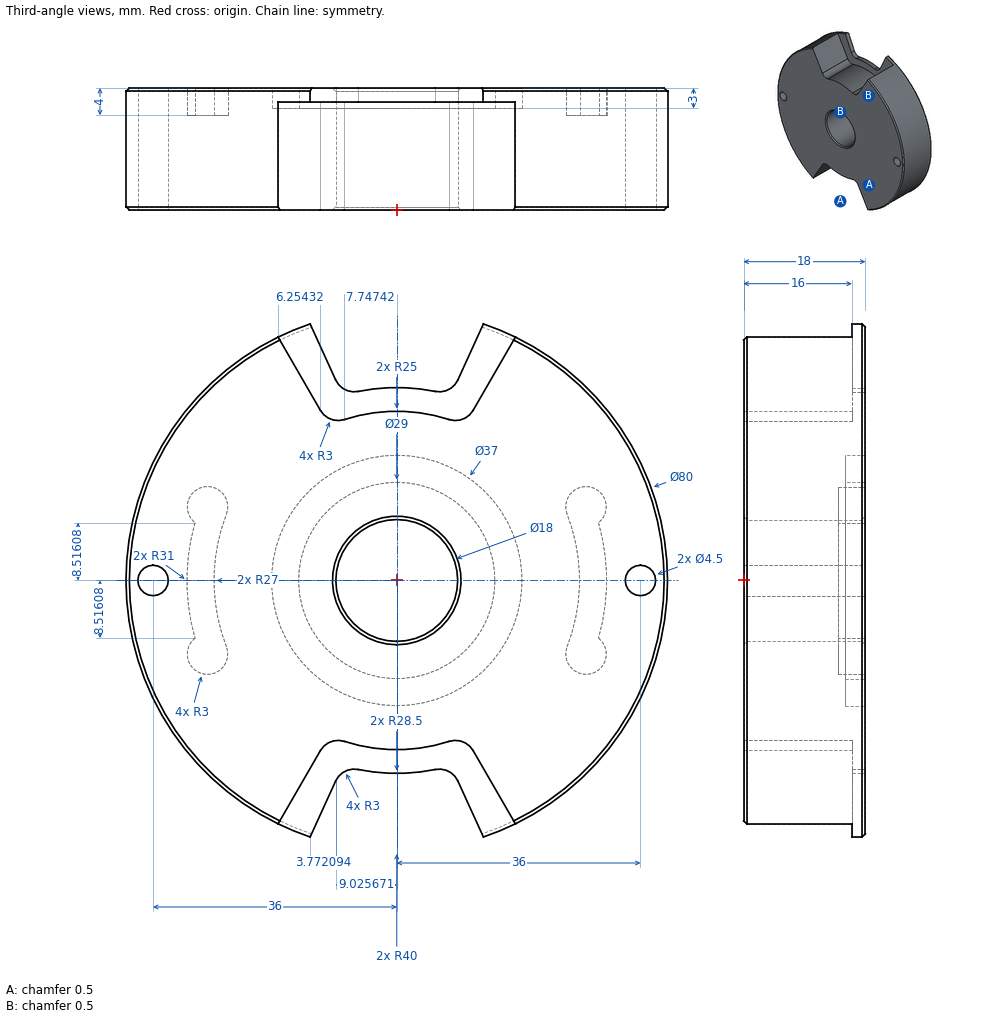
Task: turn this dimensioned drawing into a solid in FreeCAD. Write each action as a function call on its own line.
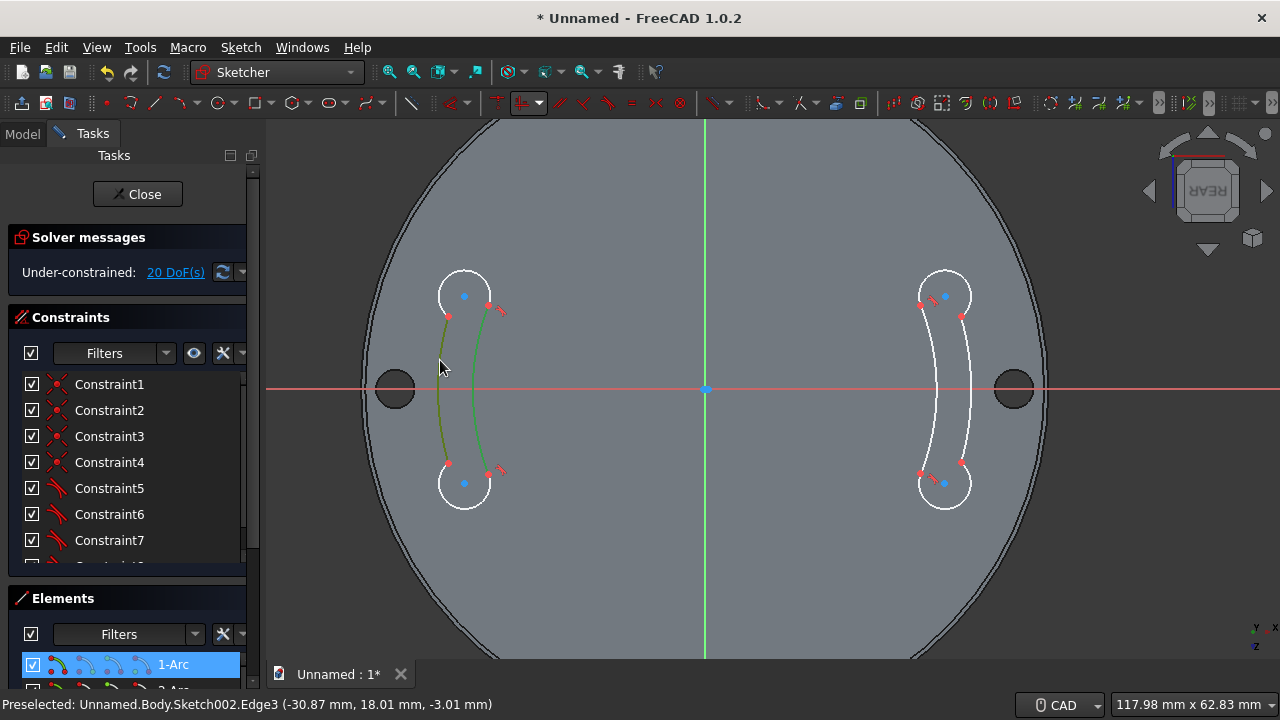
click(498, 104)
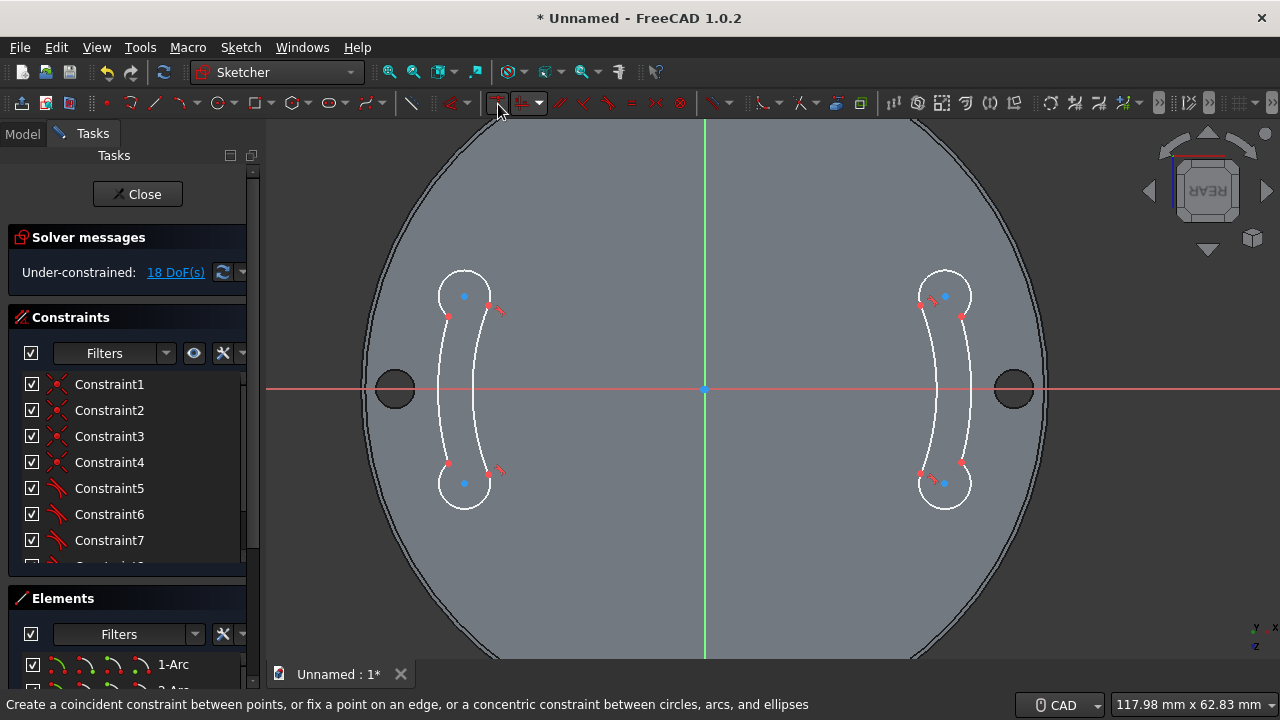
click(475, 355)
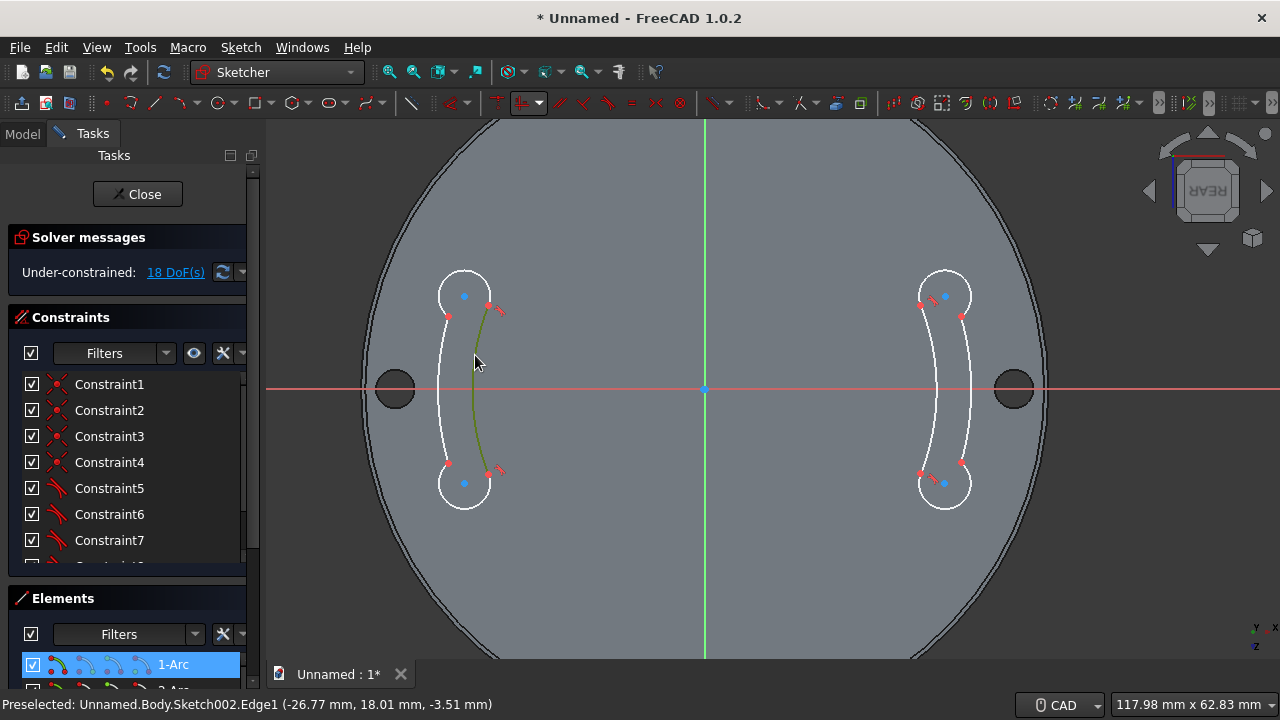
click(970, 420)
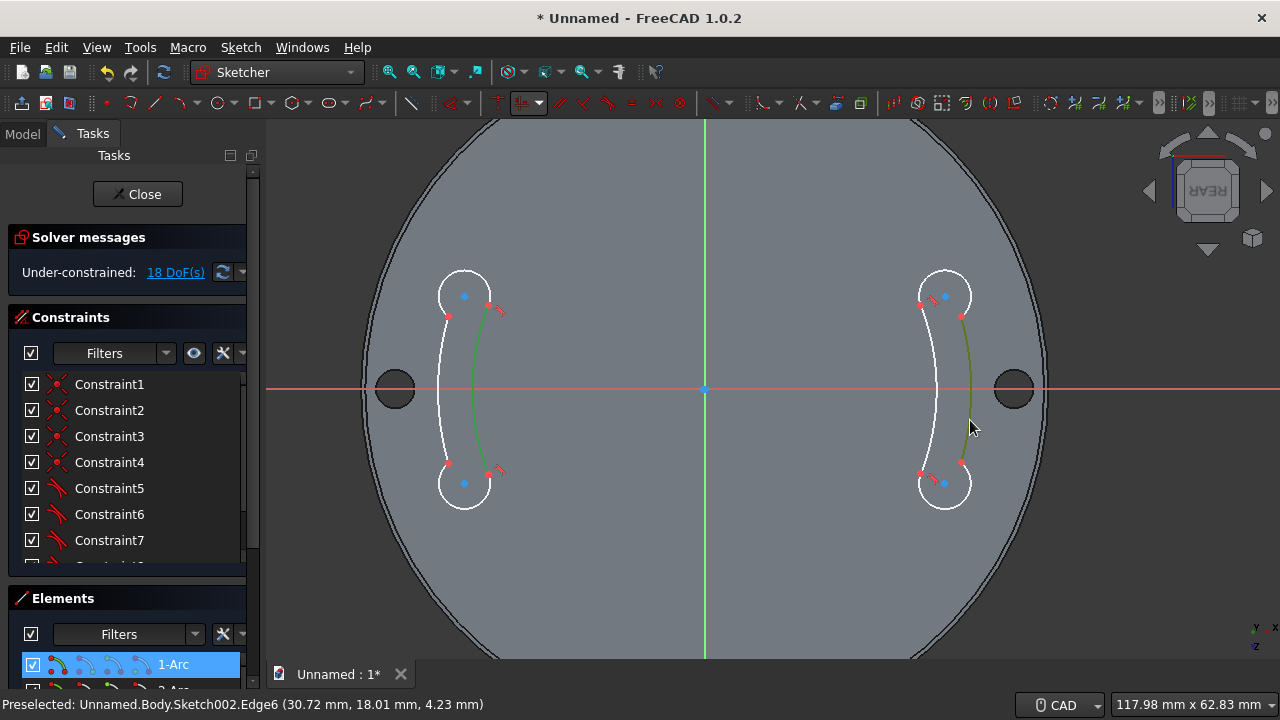
click(498, 104)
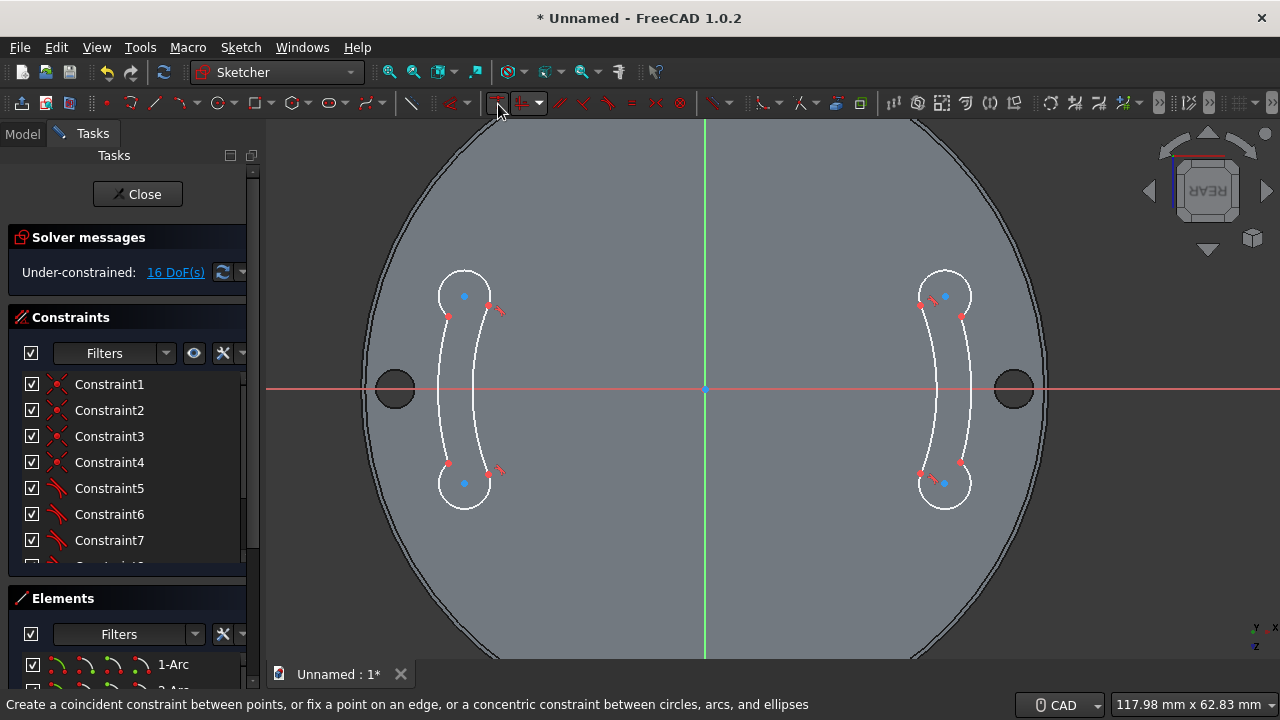
click(475, 355)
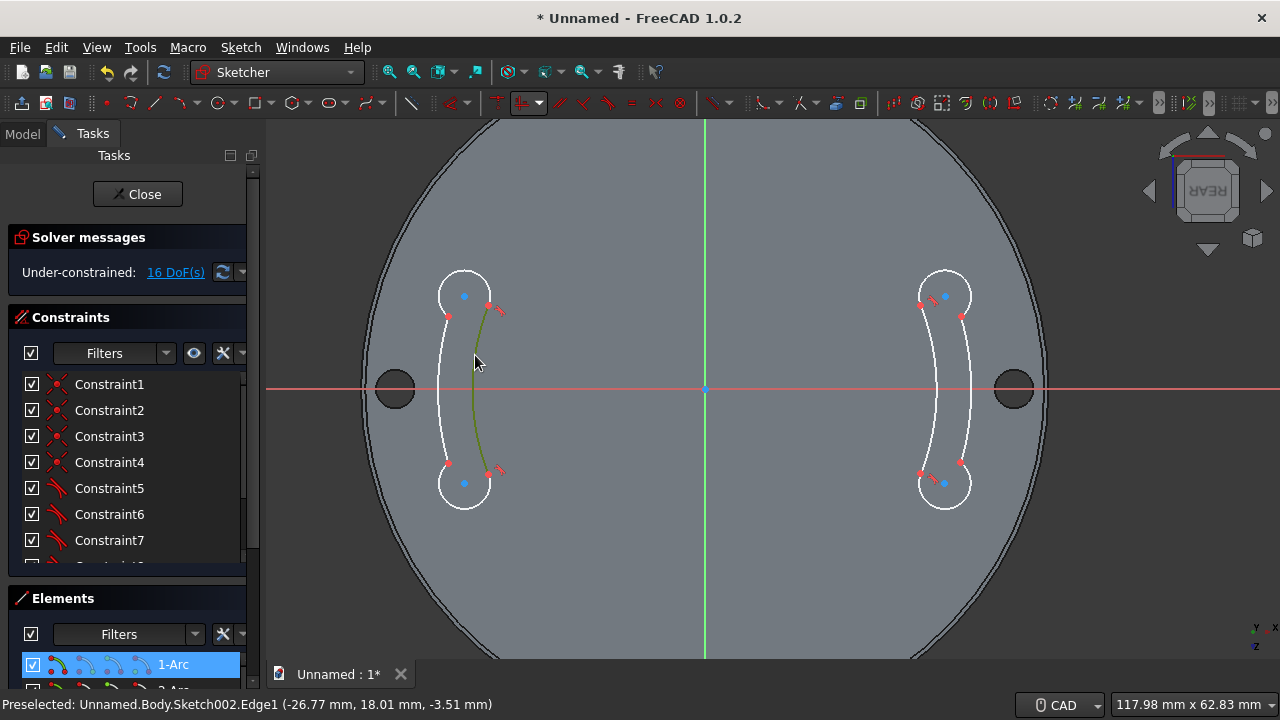
click(934, 424)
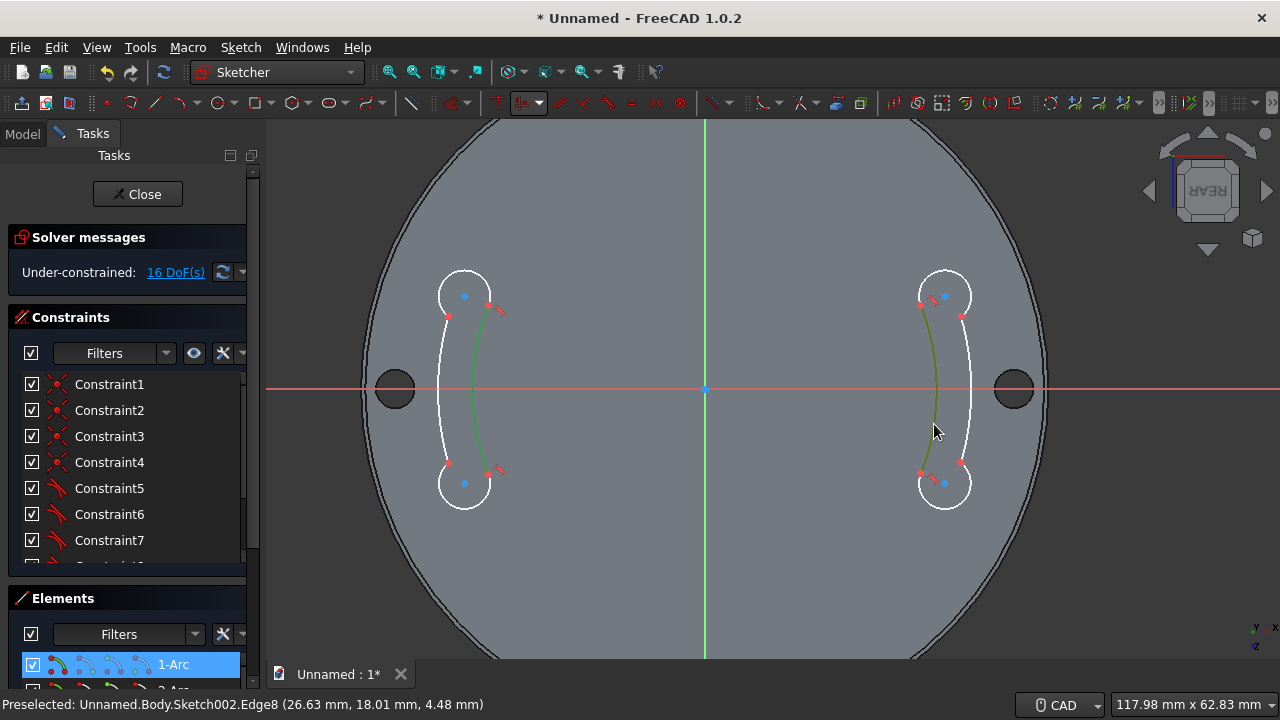
click(498, 104)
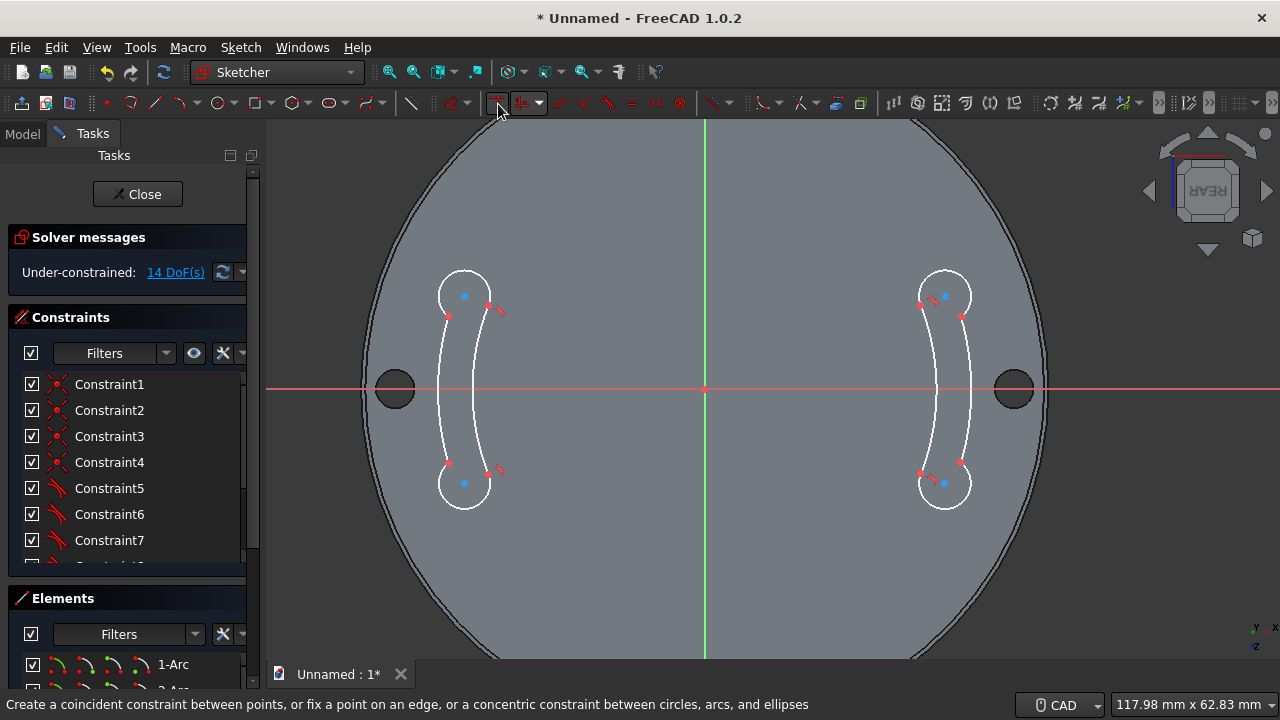
scroll(704, 389, up, 3)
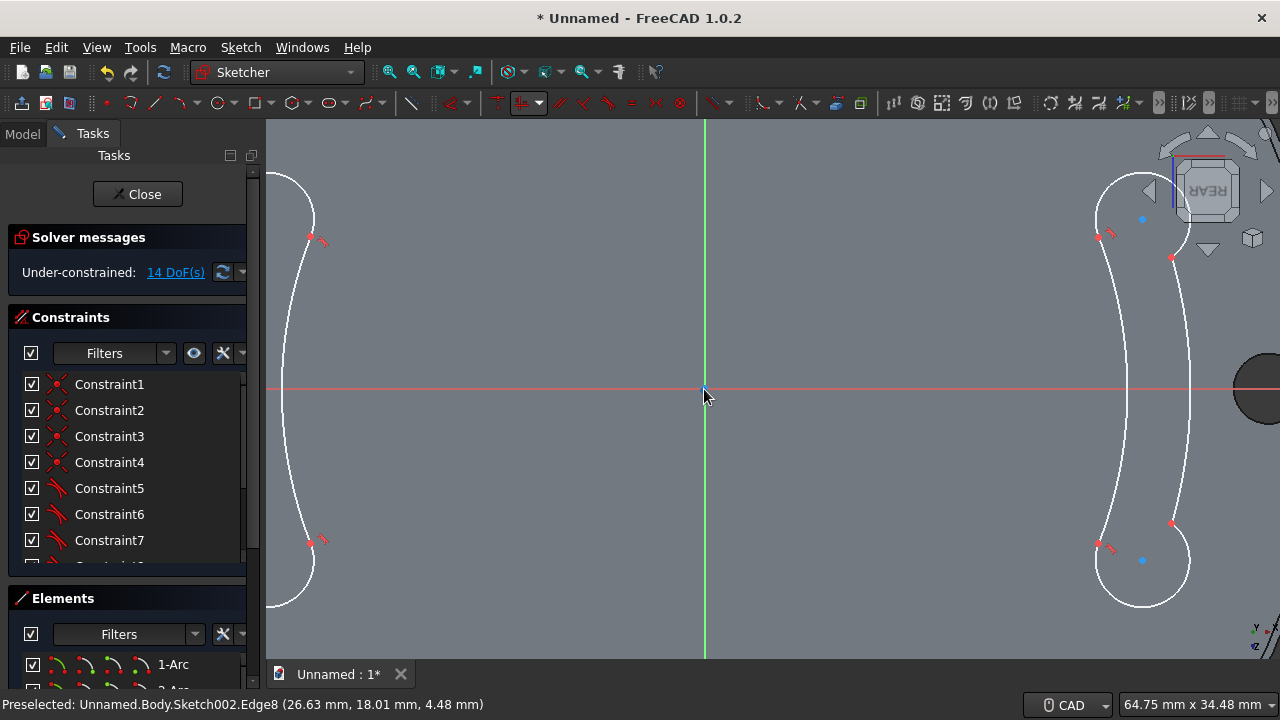
drag(694, 379, 715, 400)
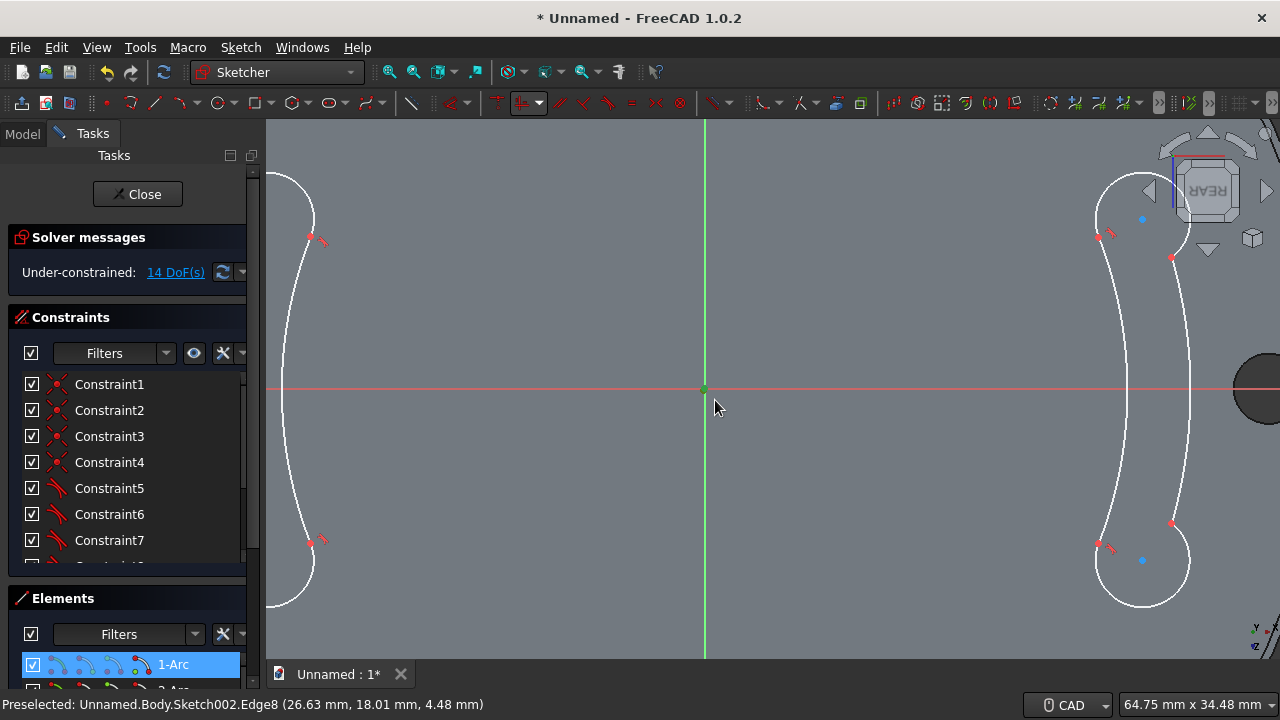
click(498, 104)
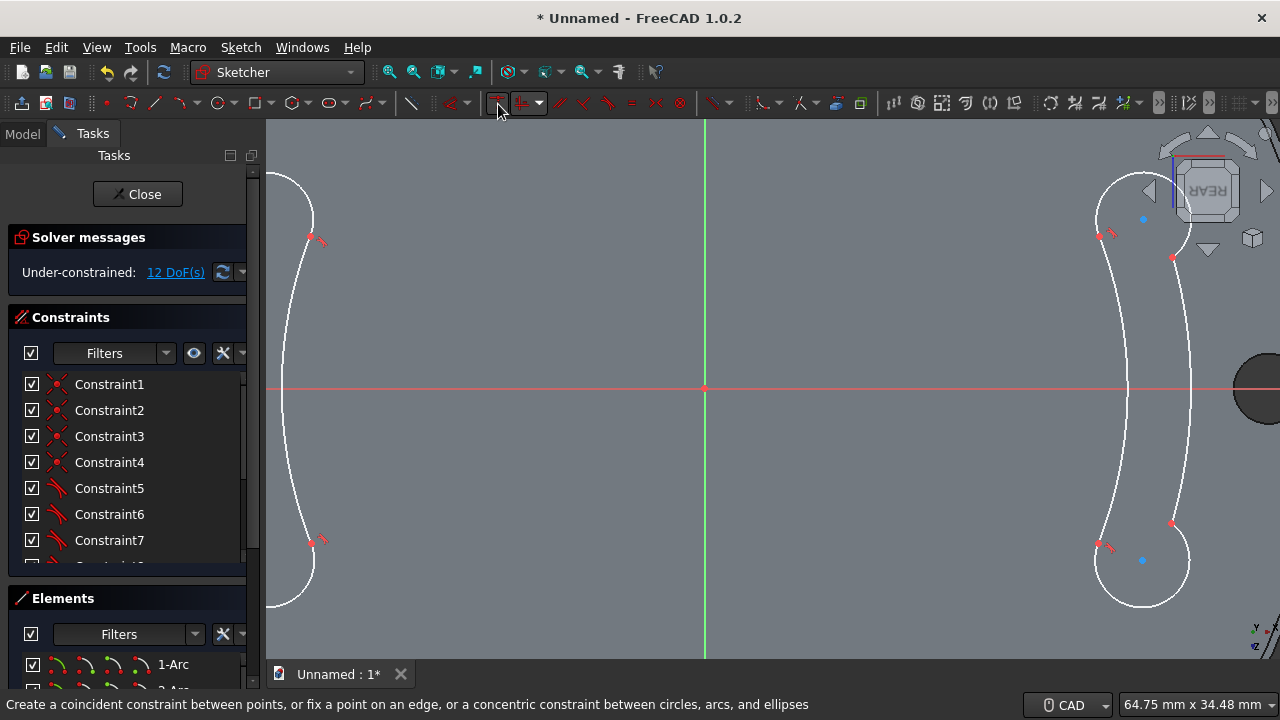
click(307, 197)